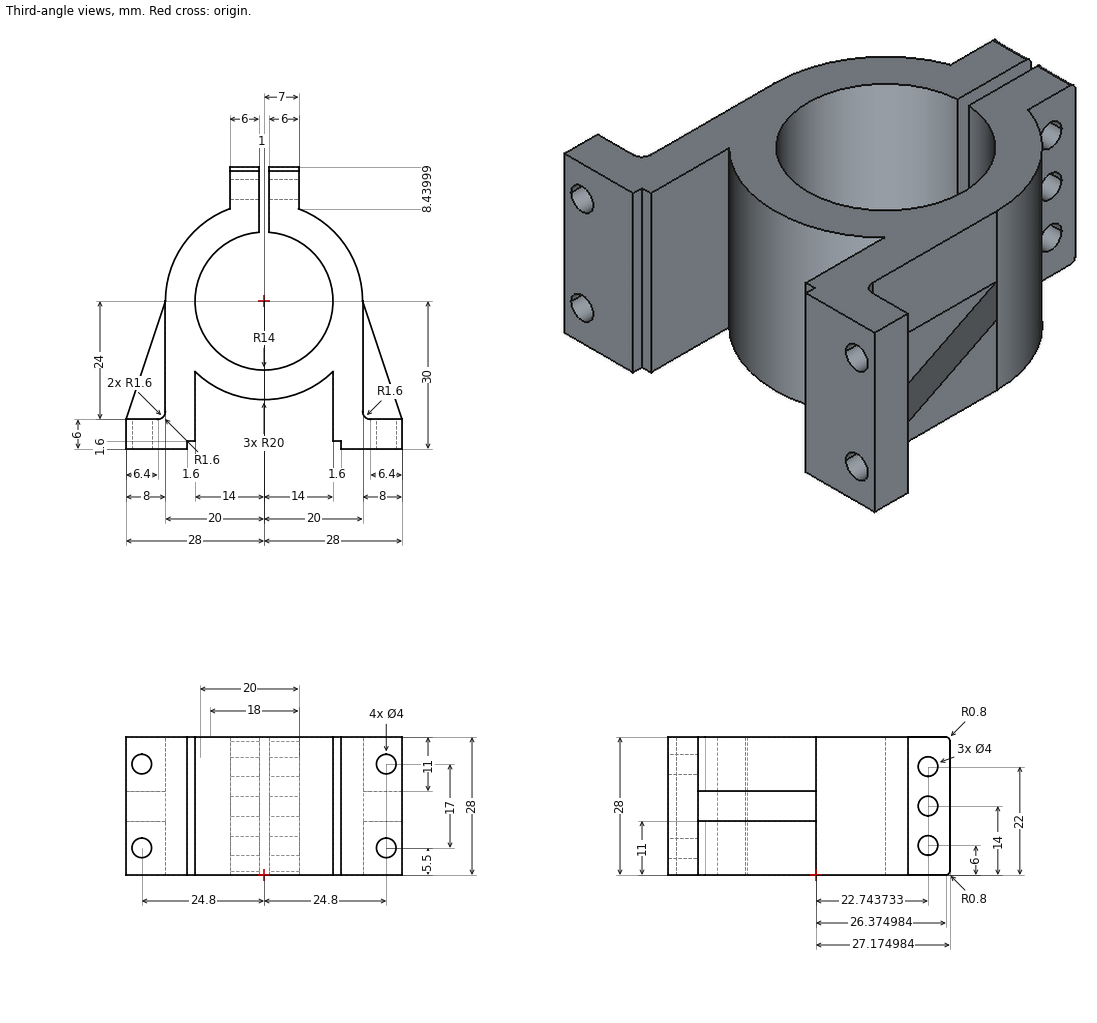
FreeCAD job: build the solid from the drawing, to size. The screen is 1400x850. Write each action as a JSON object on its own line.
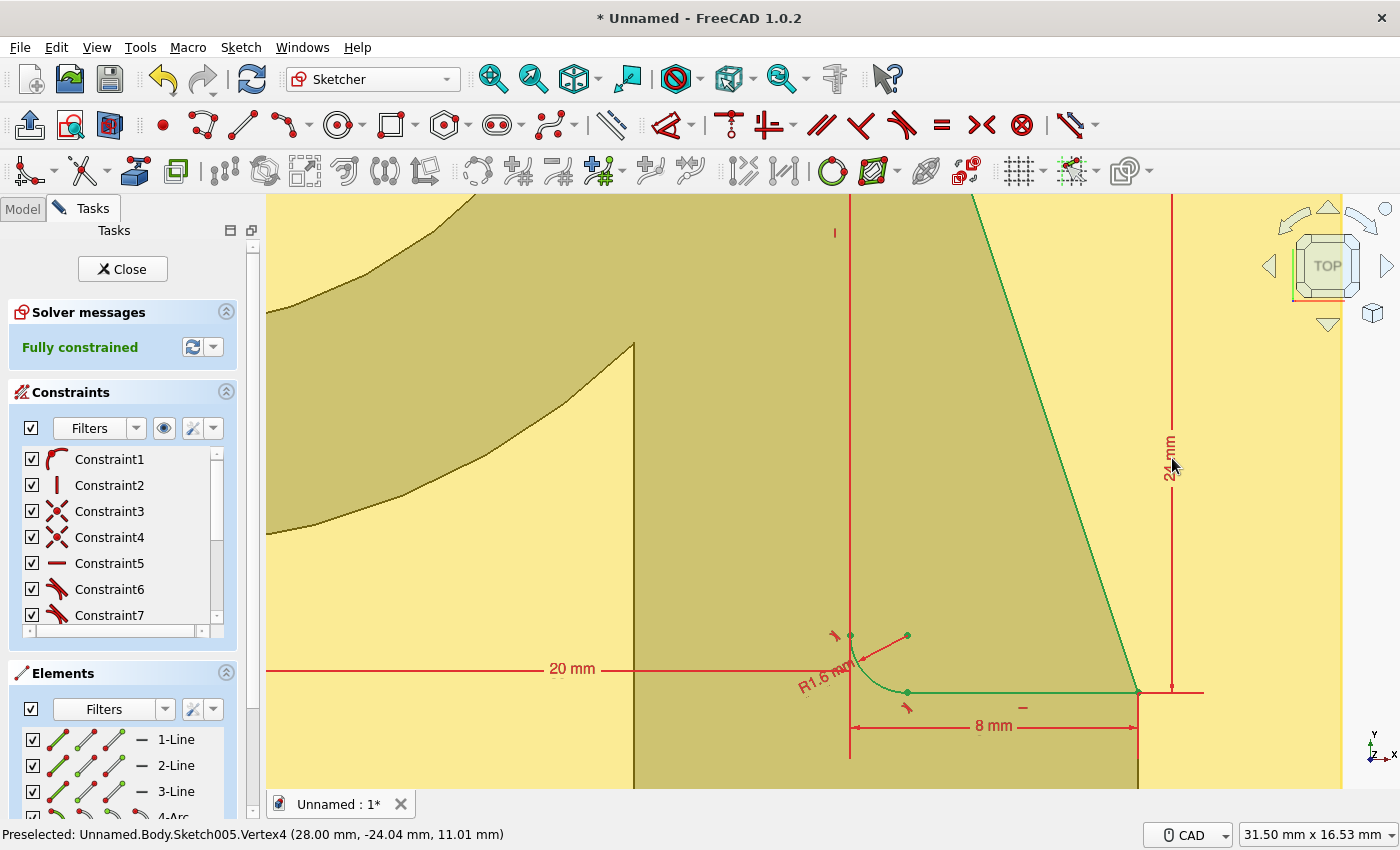
{"action": "left_click", "coordinate": [123, 269]}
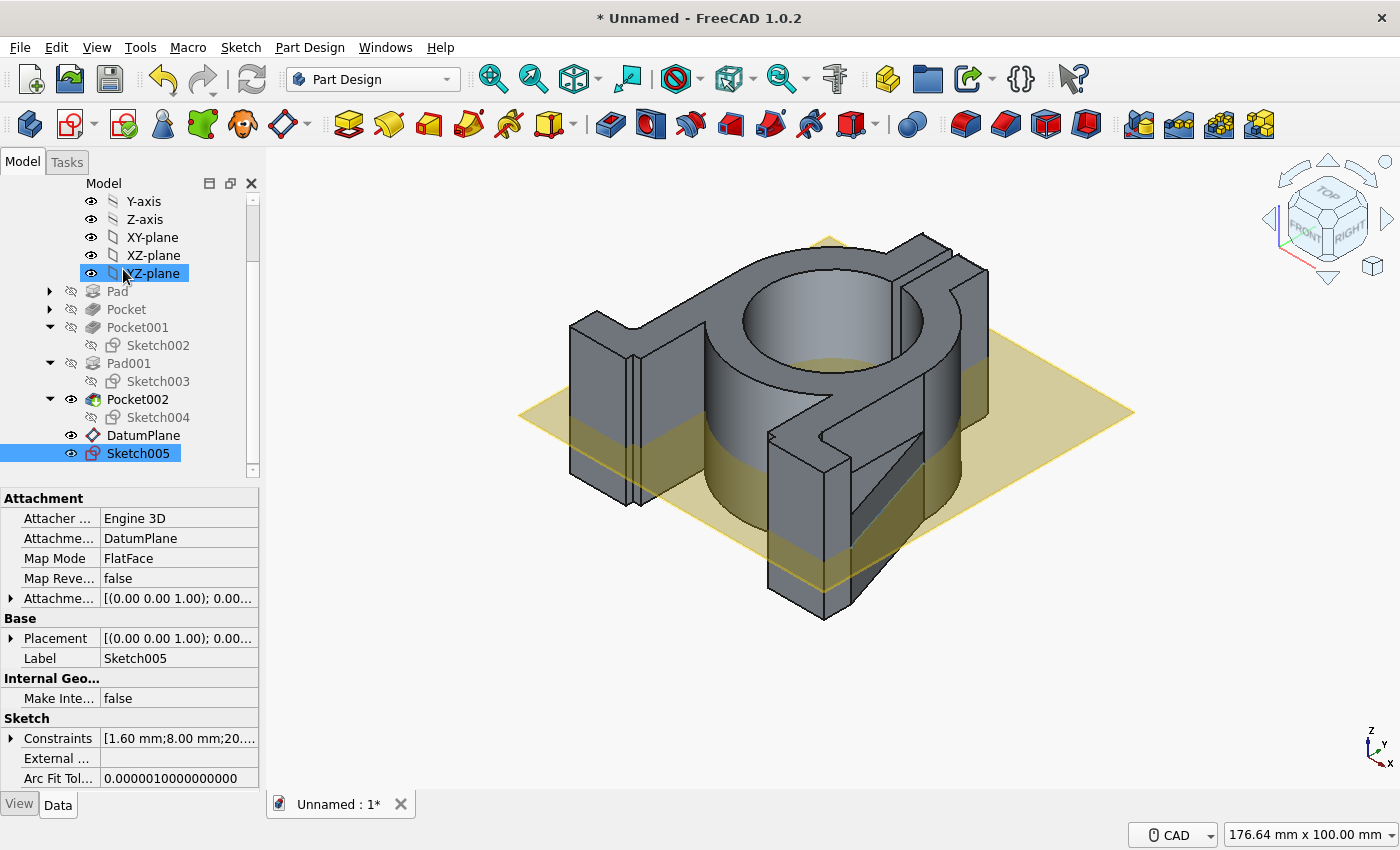
{"action": "left_click", "coordinate": [612, 124]}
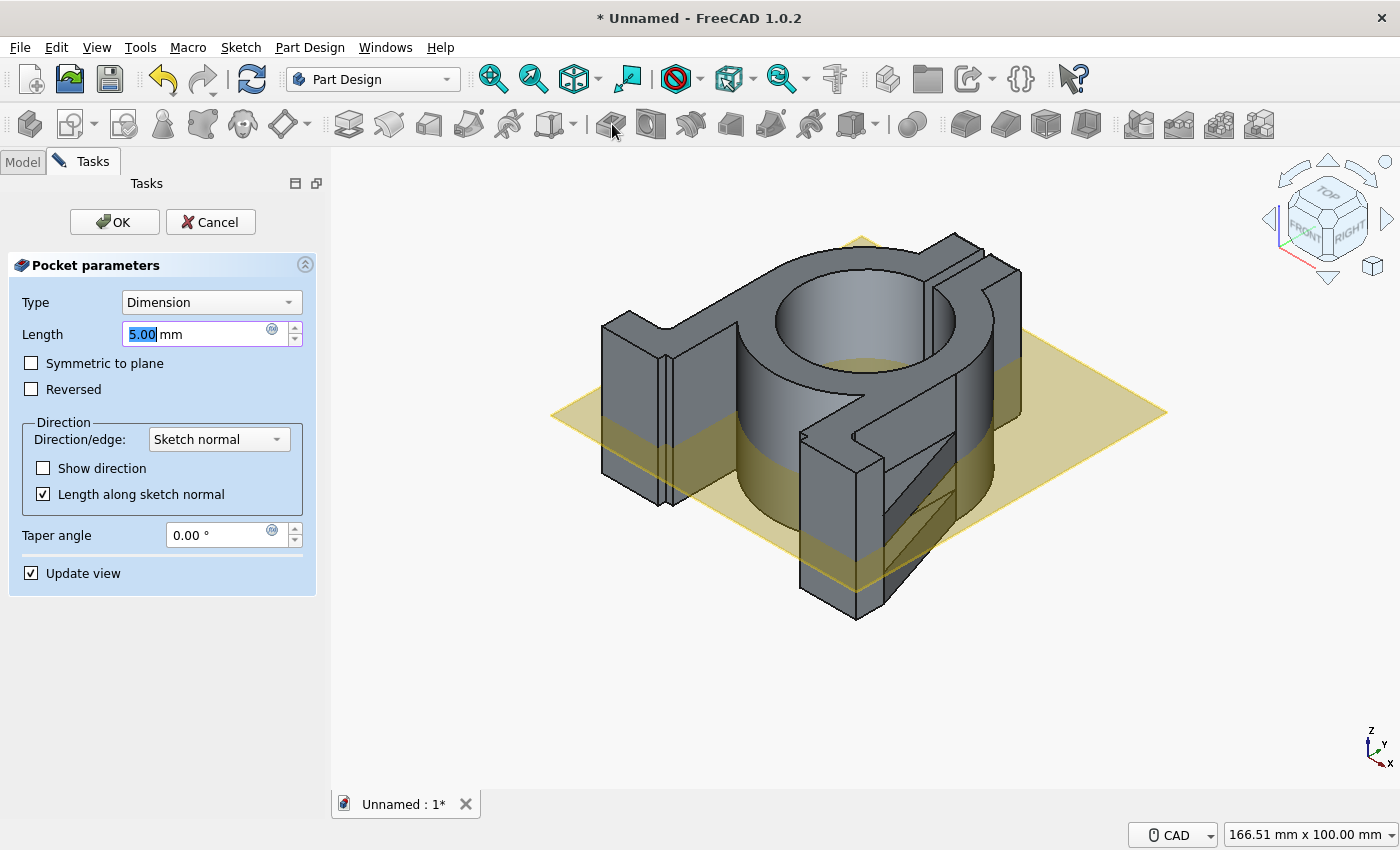
{"action": "type", "text": "11"}
{"action": "key", "text": "Tab"}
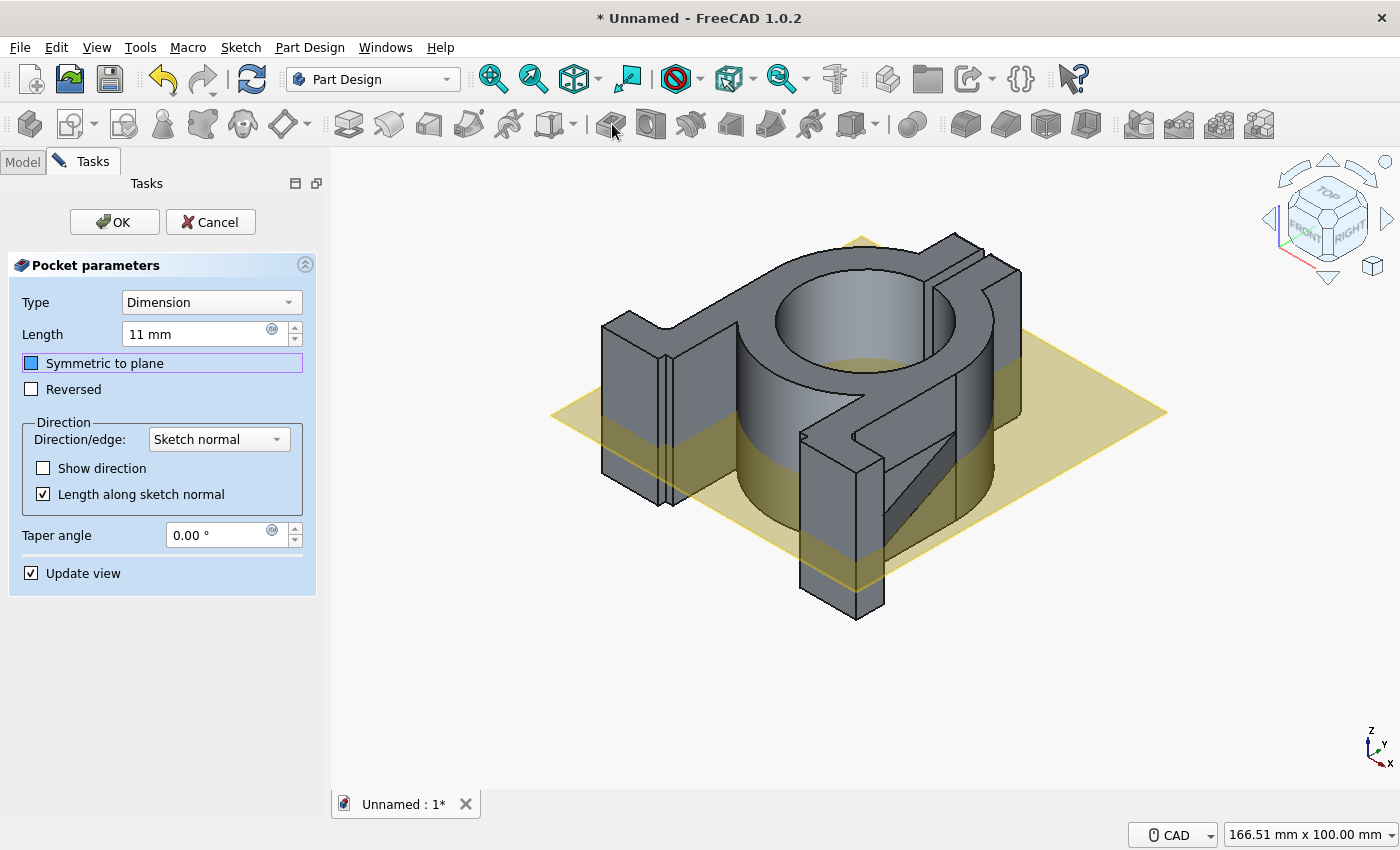
{"action": "left_click", "coordinate": [115, 222]}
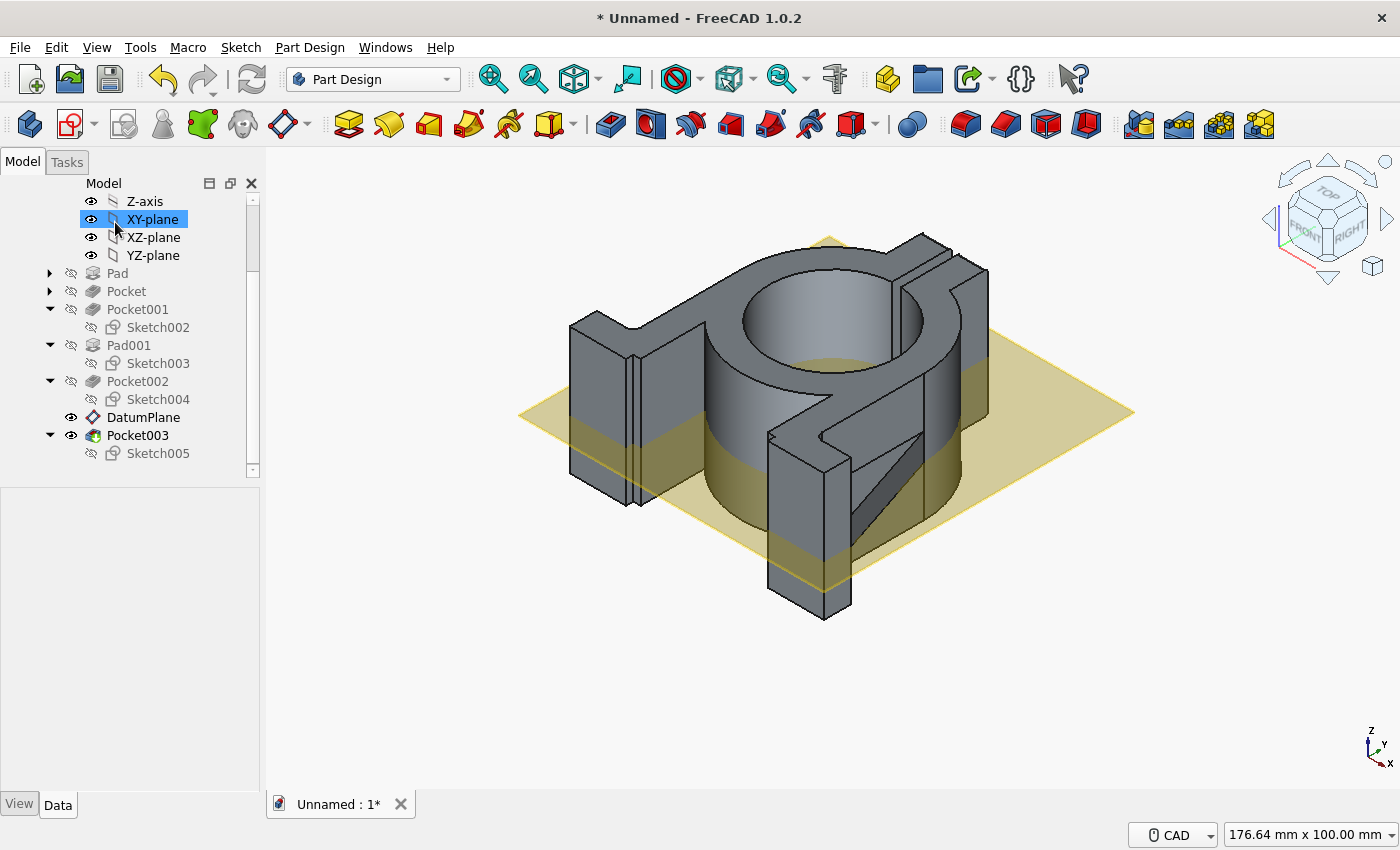
{"action": "left_click", "coordinate": [116, 417]}
{"action": "key", "text": "space"}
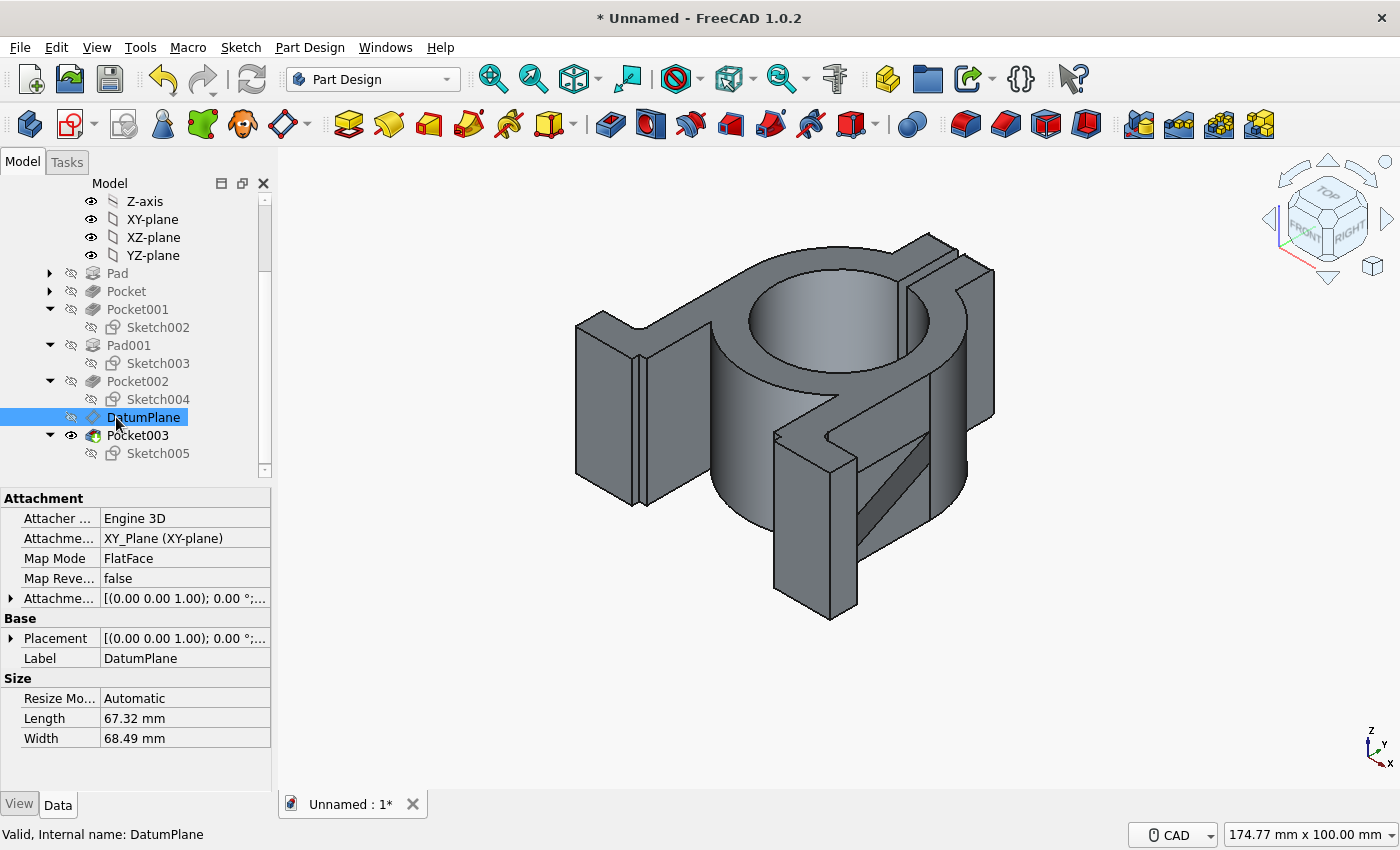
{"action": "key", "text": "5"}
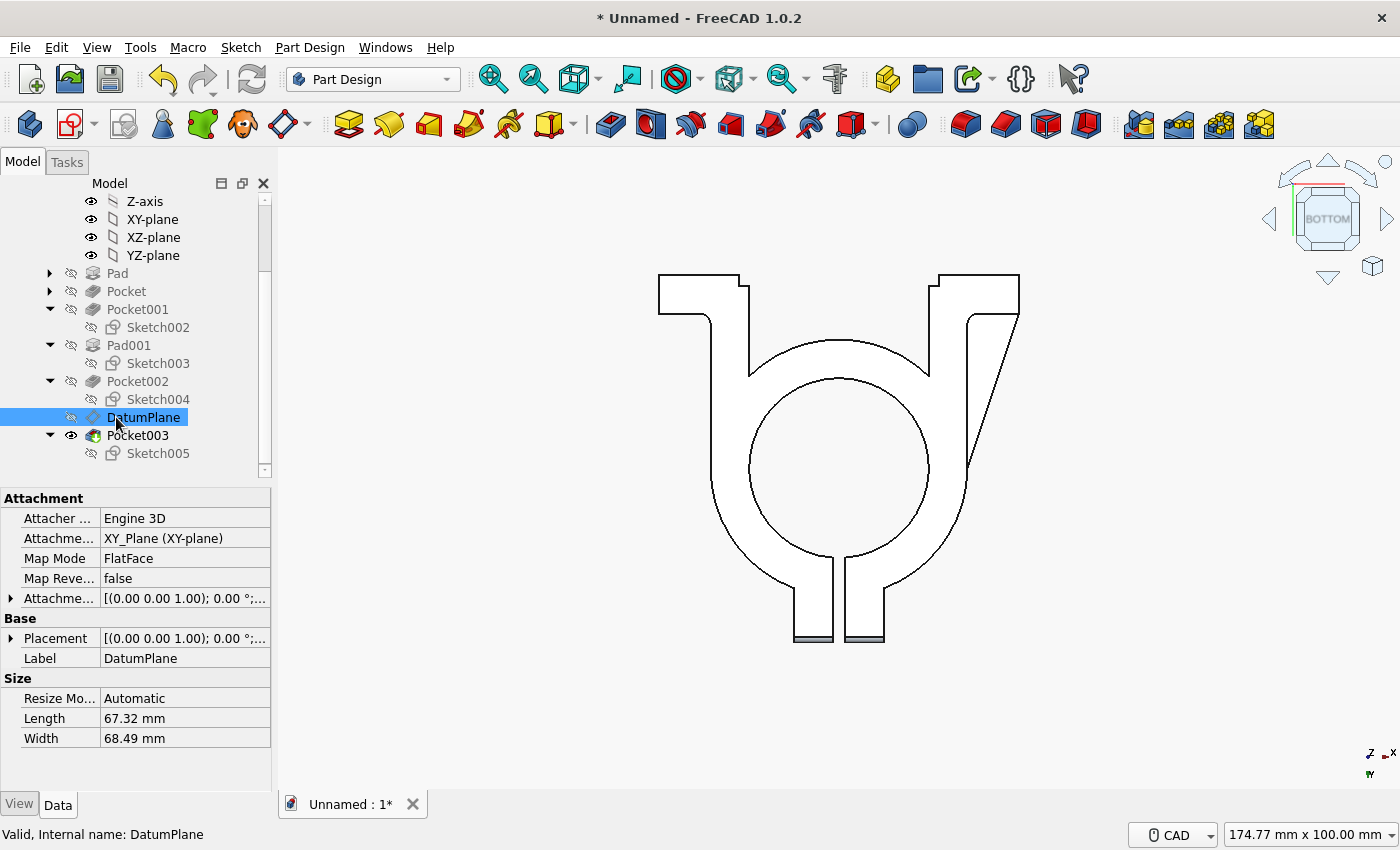
{"action": "left_click", "coordinate": [736, 404]}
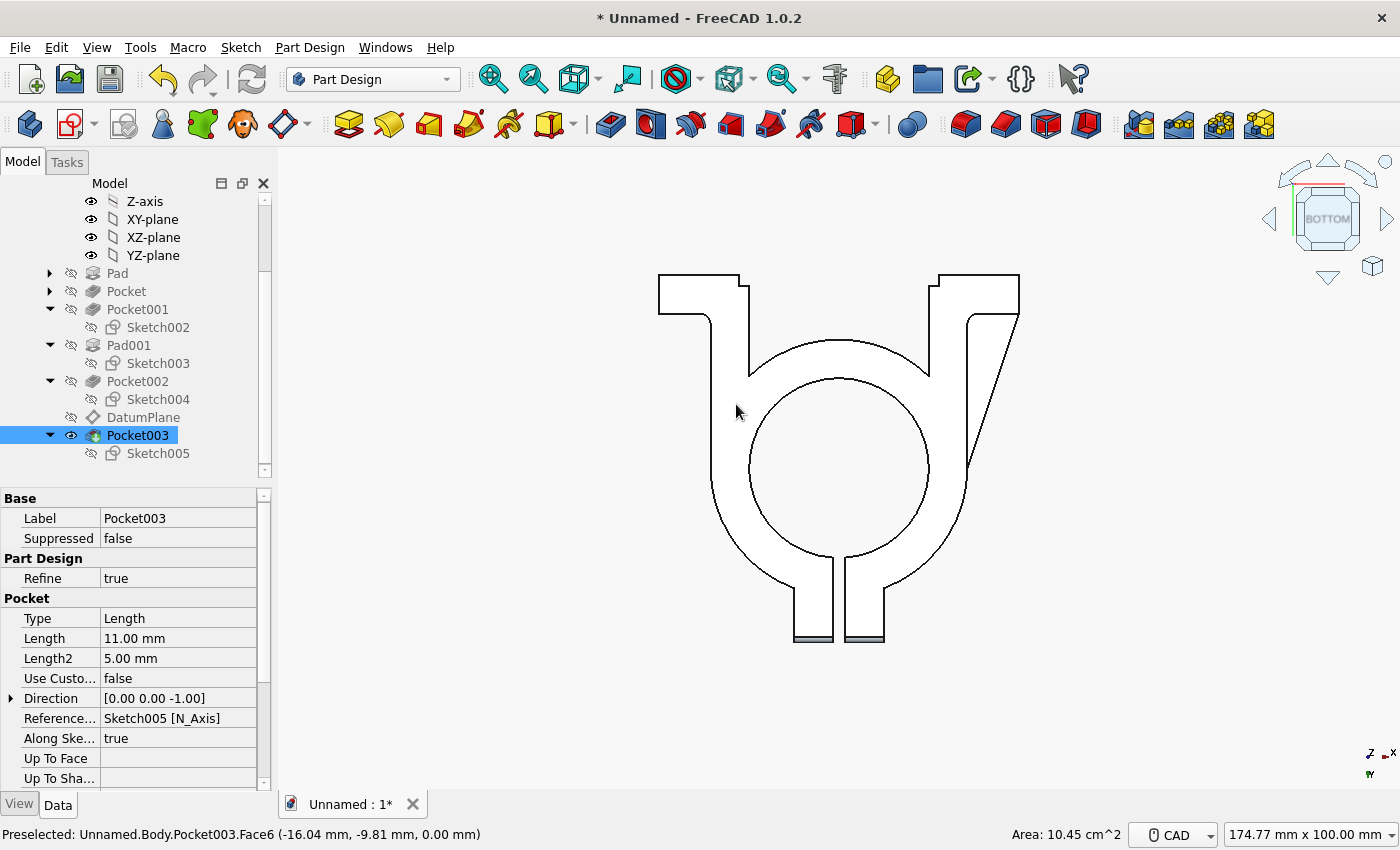
{"action": "left_click", "coordinate": [70, 124]}